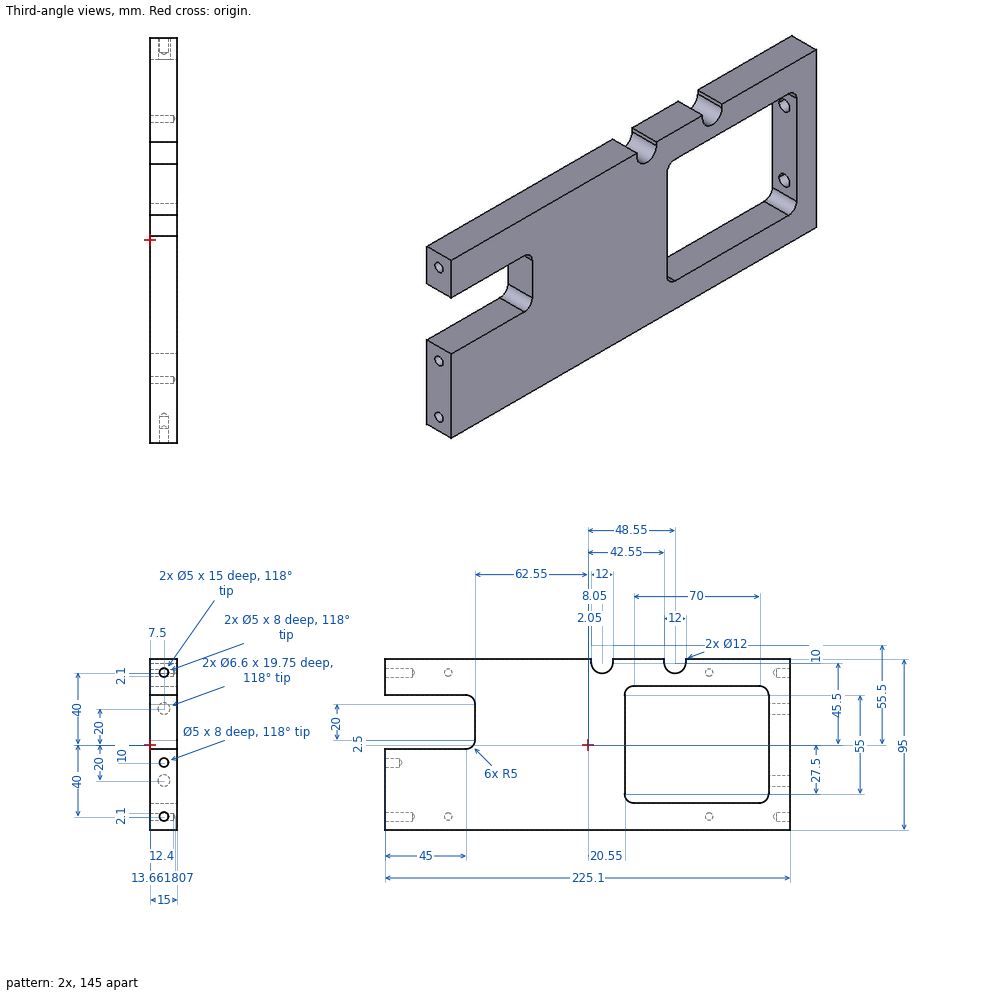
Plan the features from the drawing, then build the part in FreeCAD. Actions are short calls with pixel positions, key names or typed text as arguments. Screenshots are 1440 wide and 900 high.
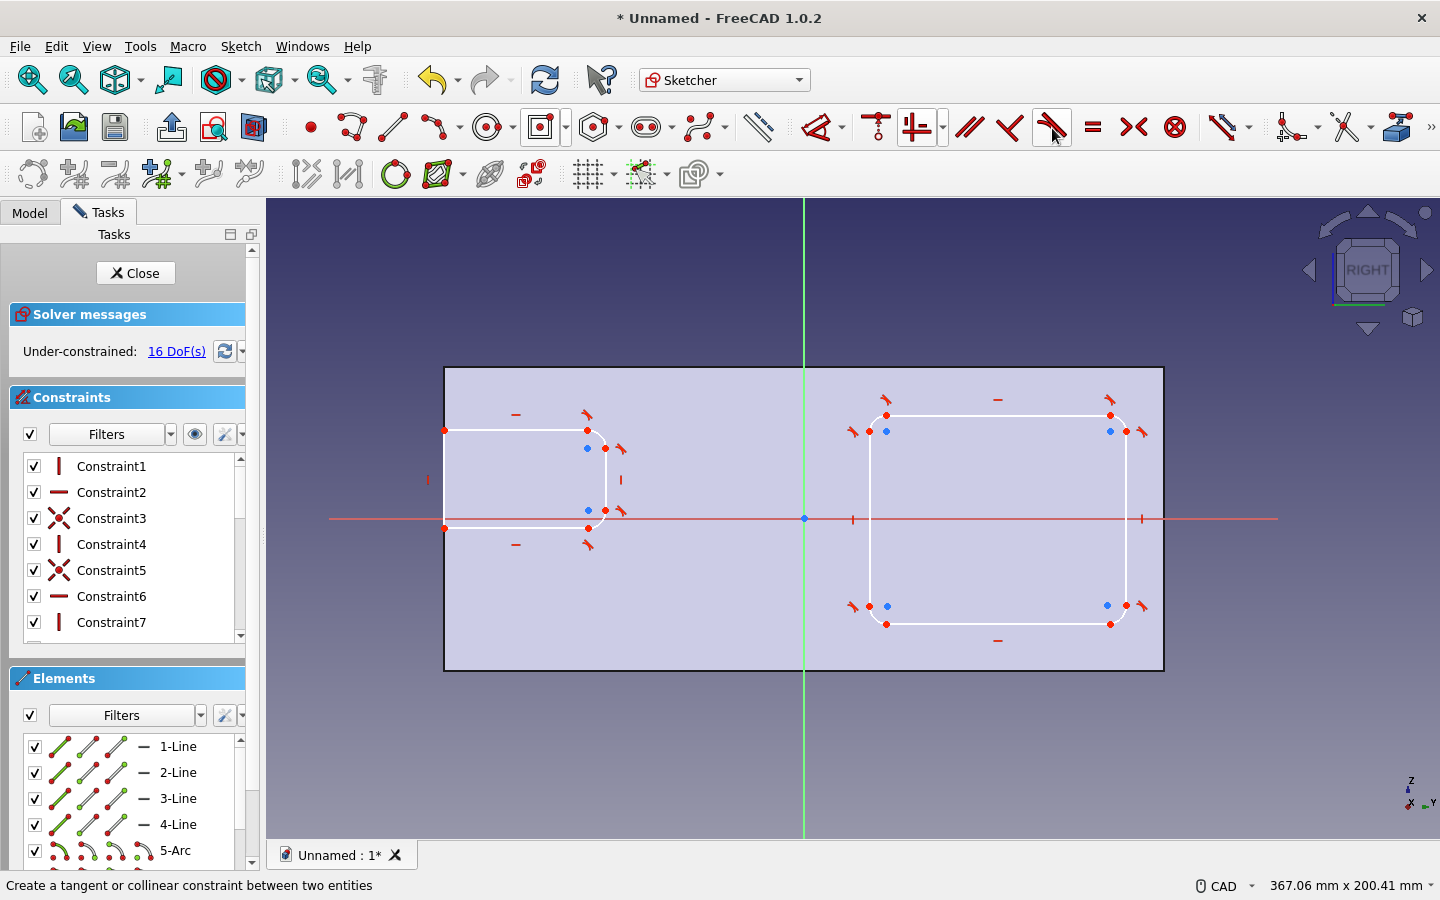
click(1043, 624)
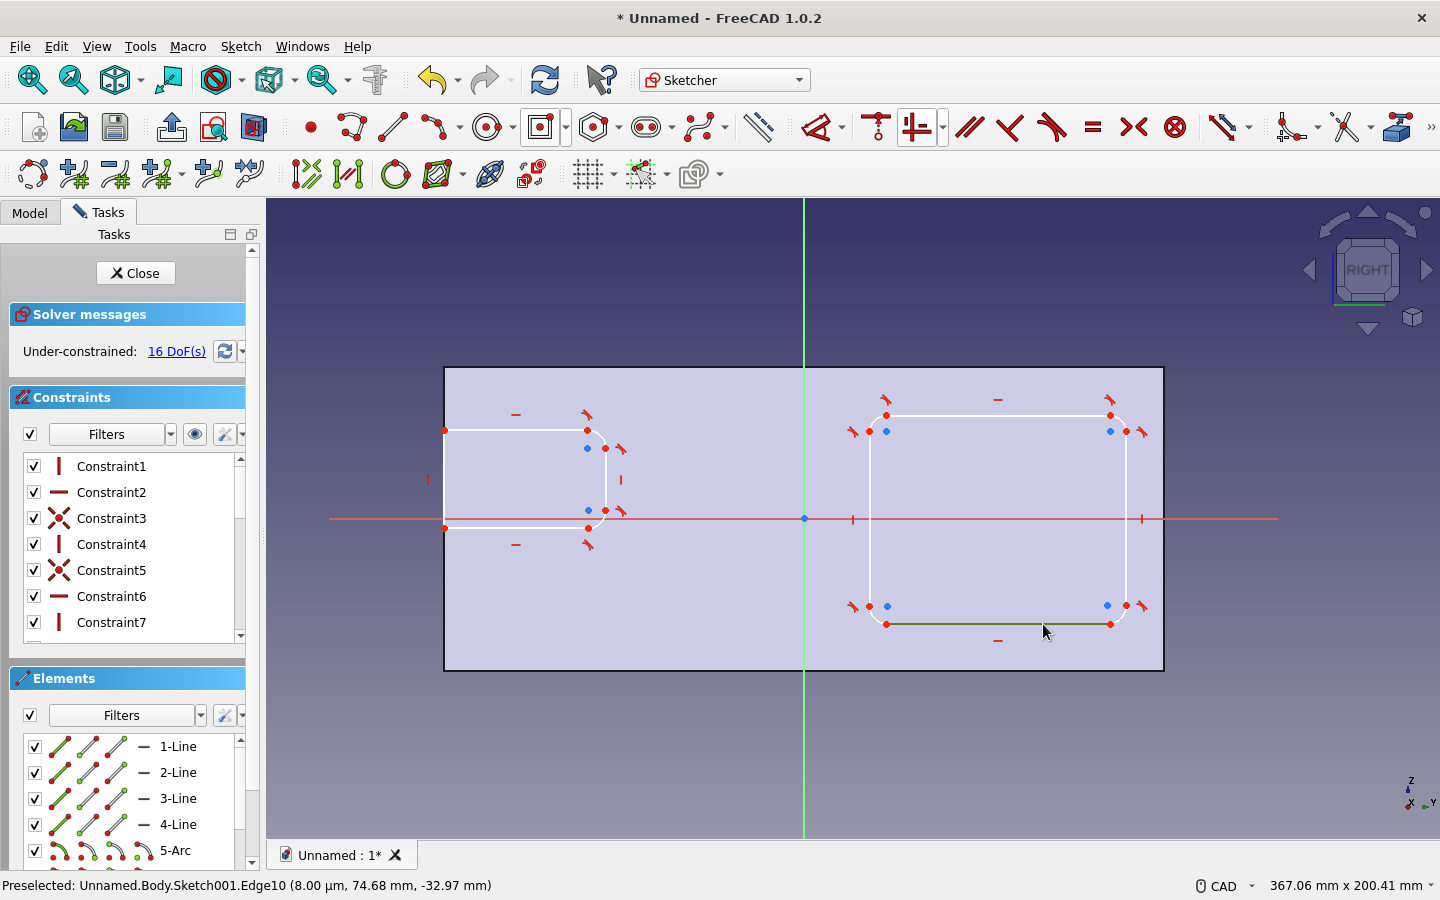
click(1122, 618)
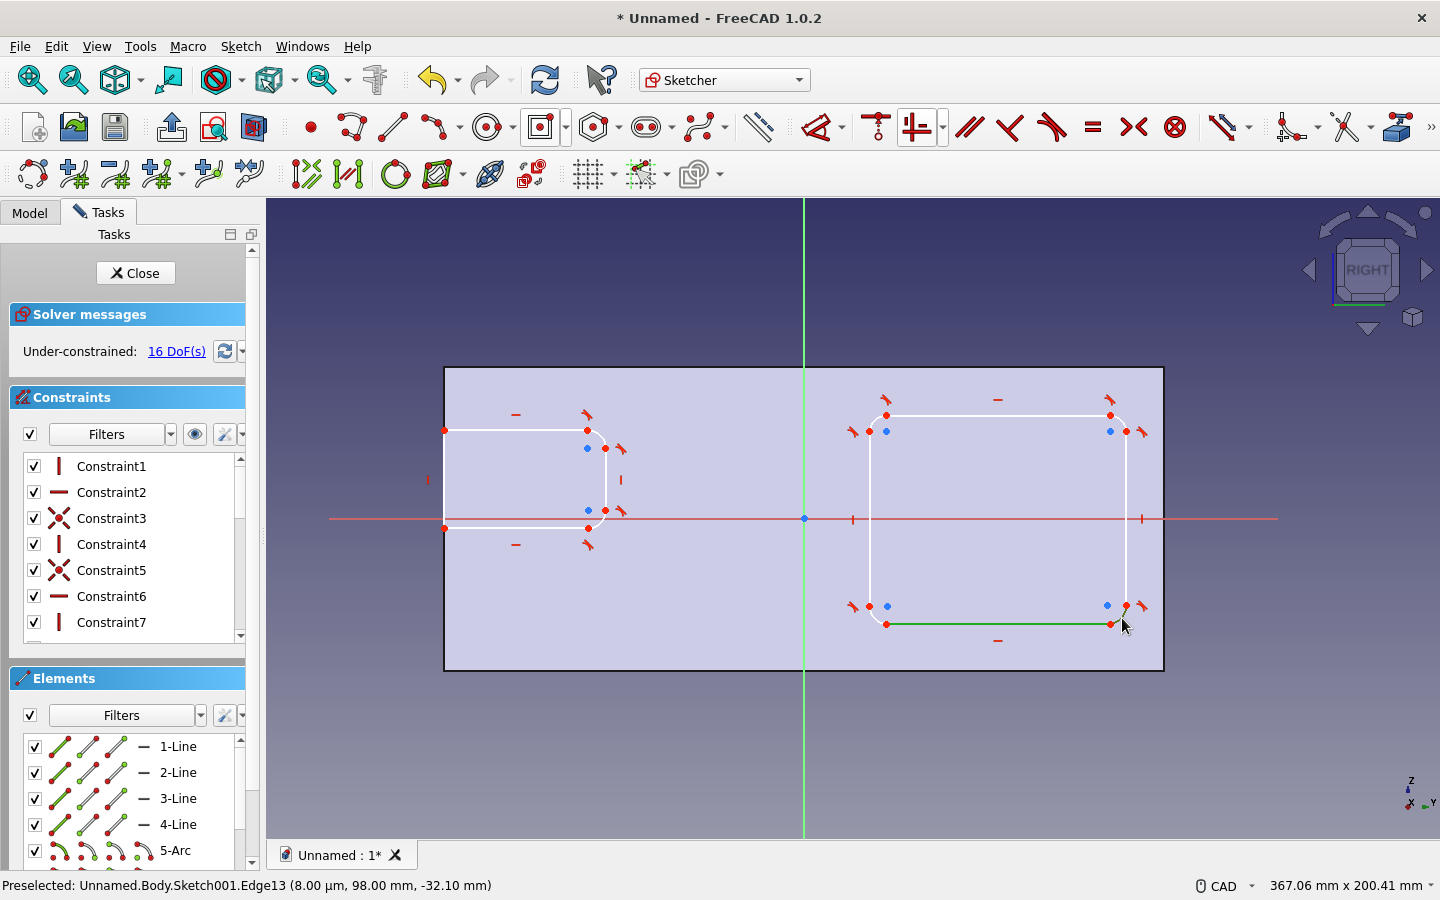
click(1052, 128)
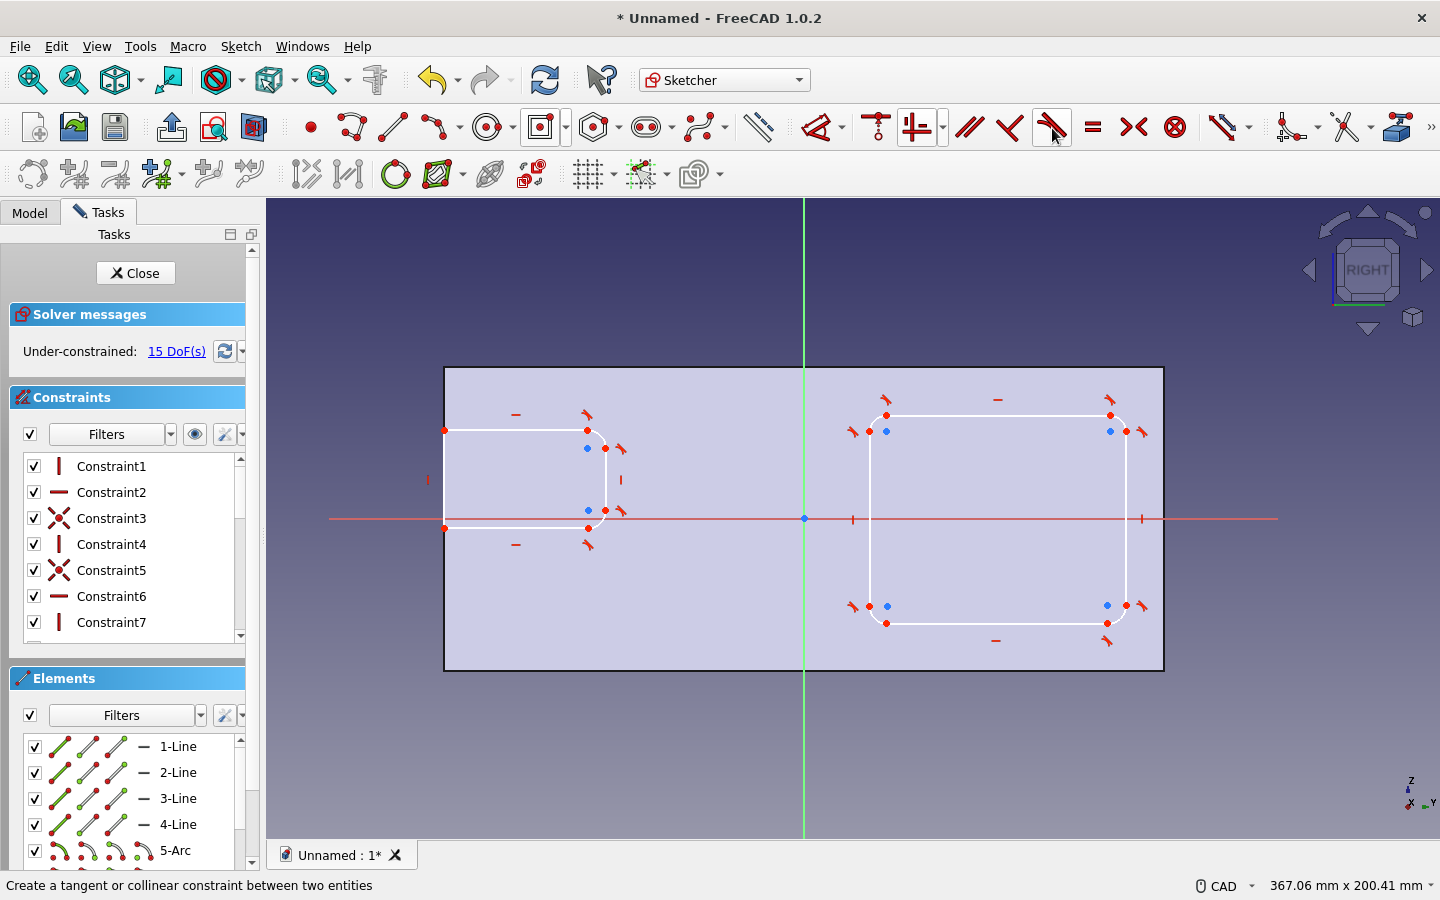
click(1041, 624)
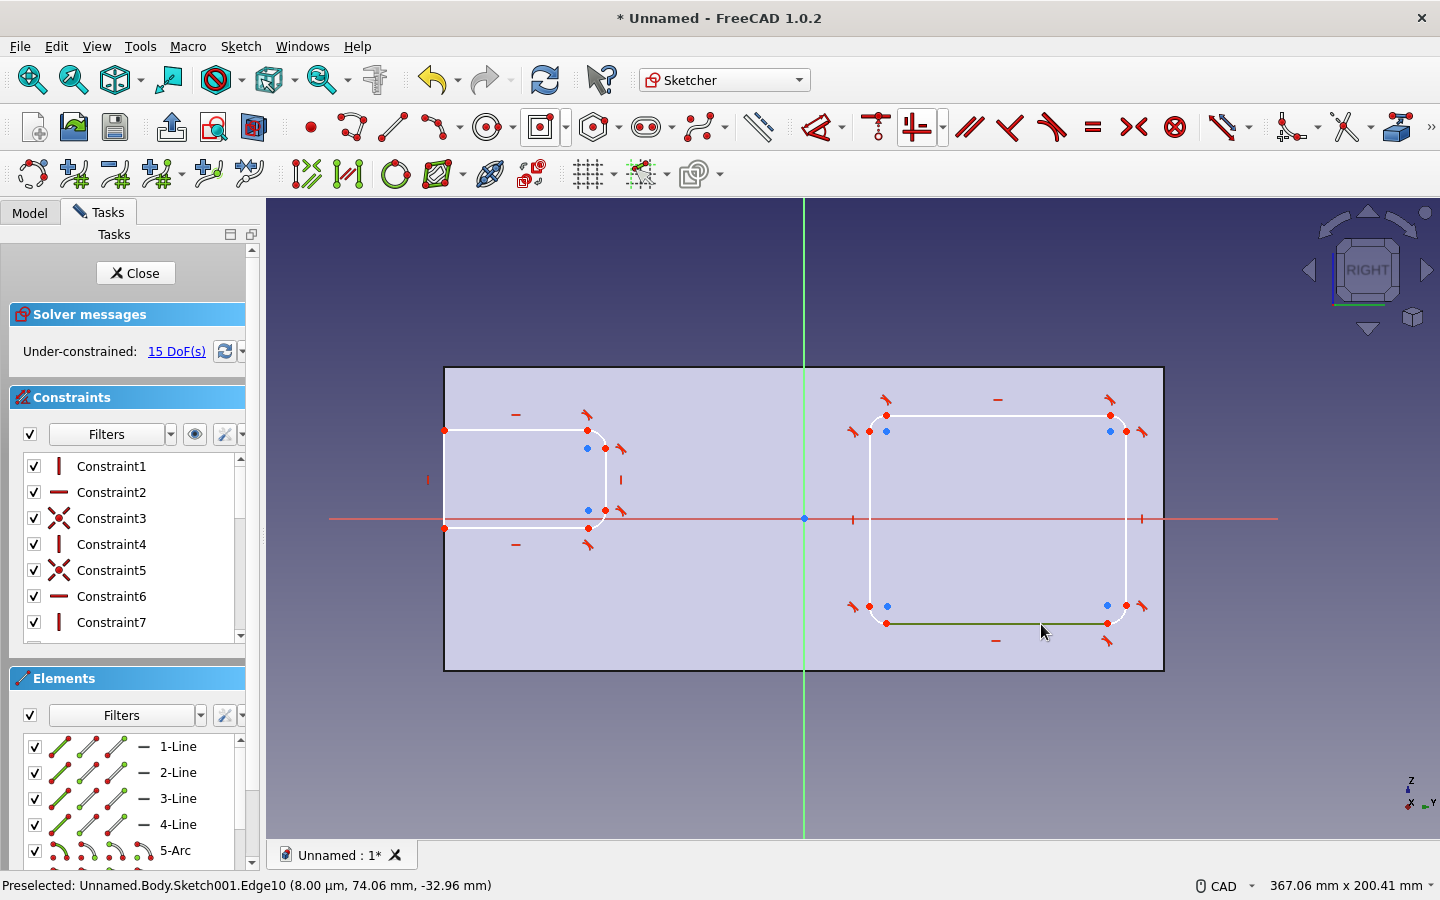
click(875, 618)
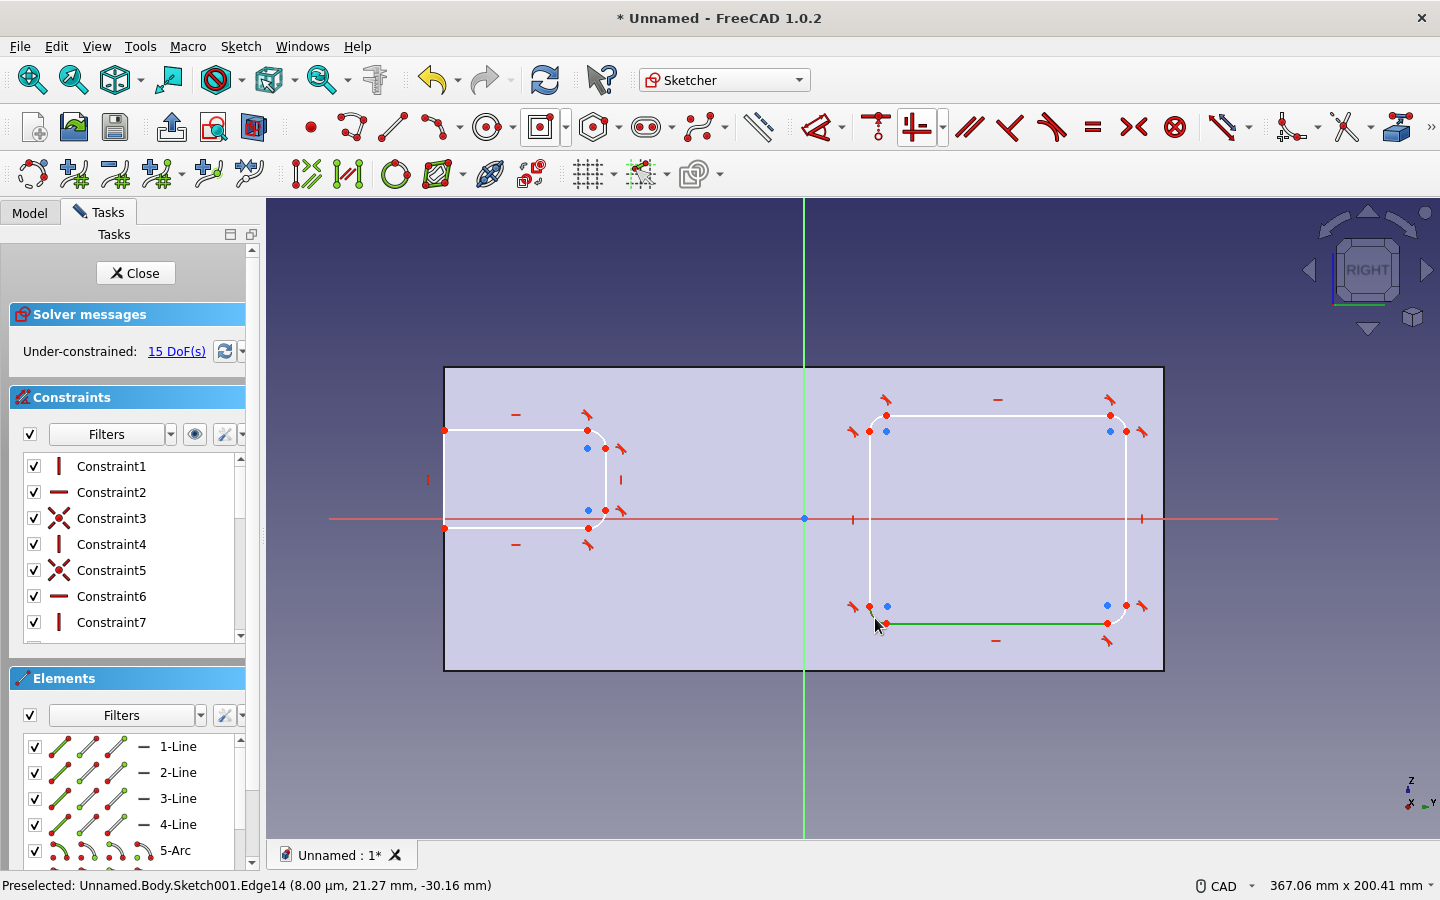
click(1052, 128)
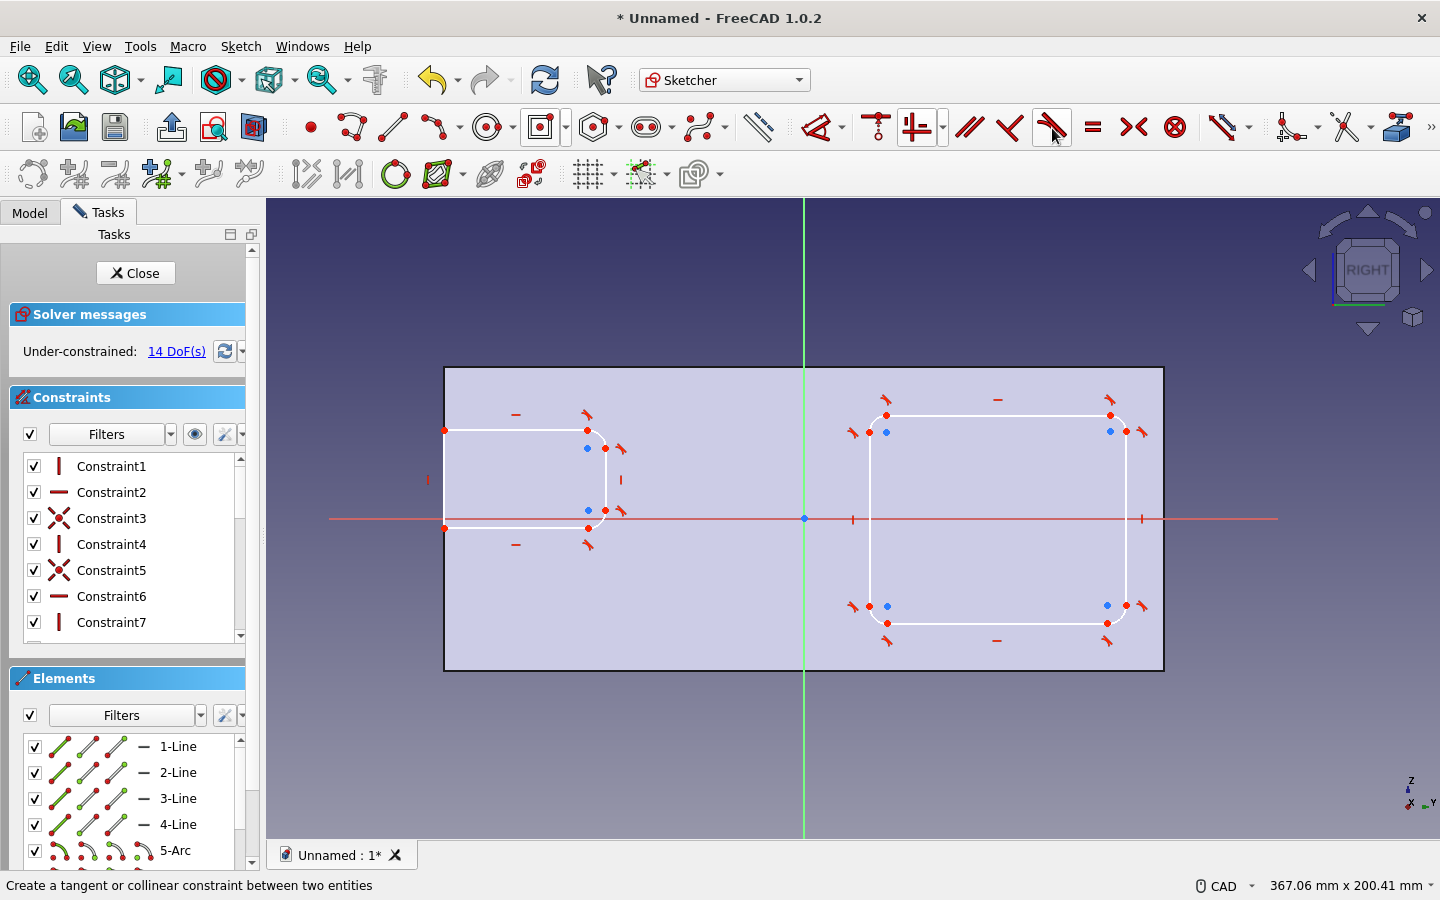
scroll(604, 519, up, 3)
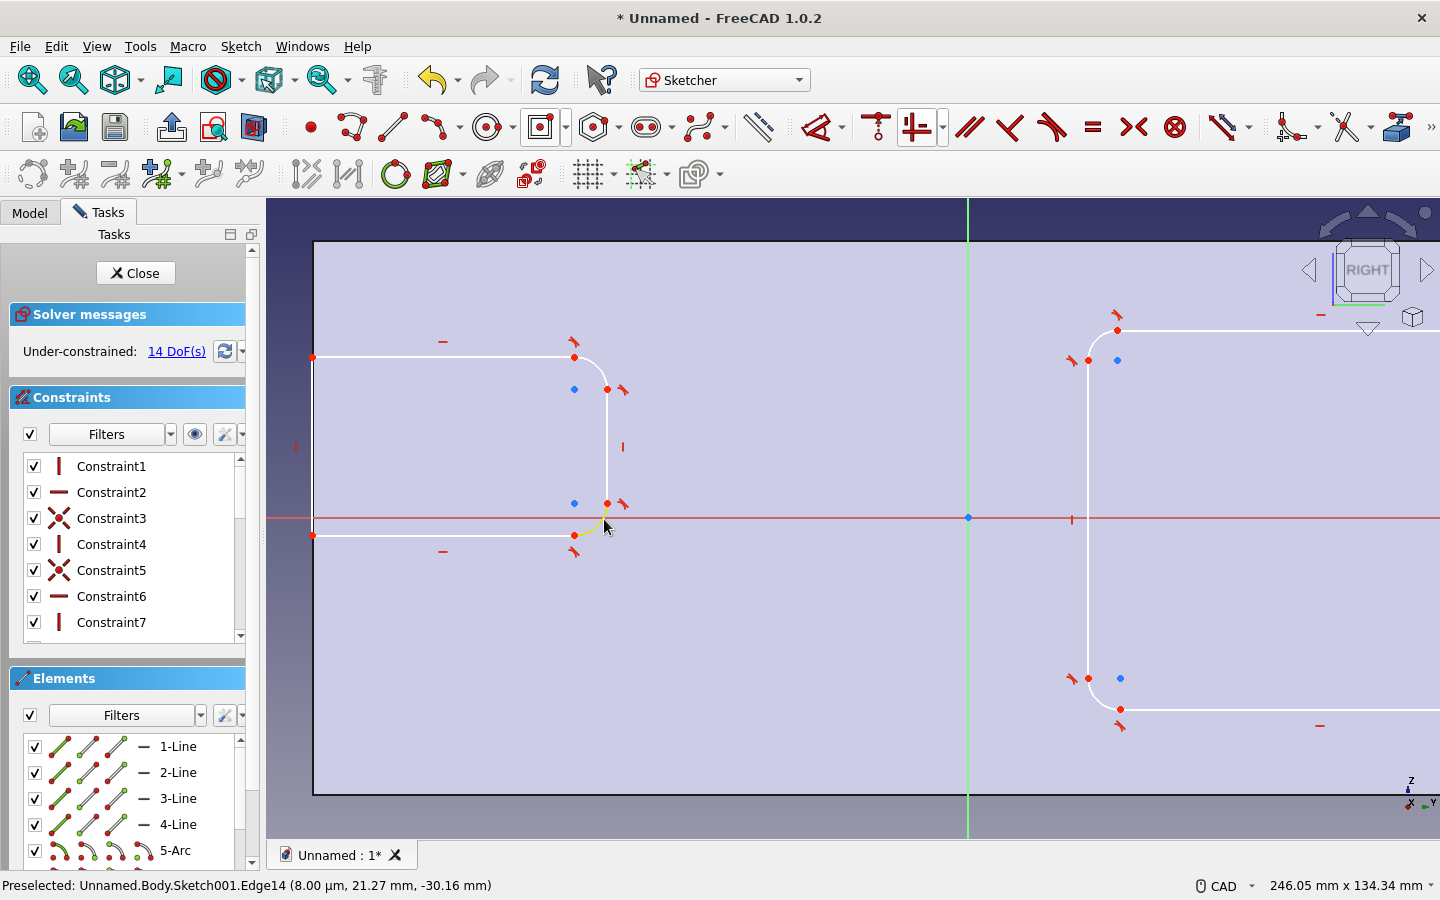
click(604, 518)